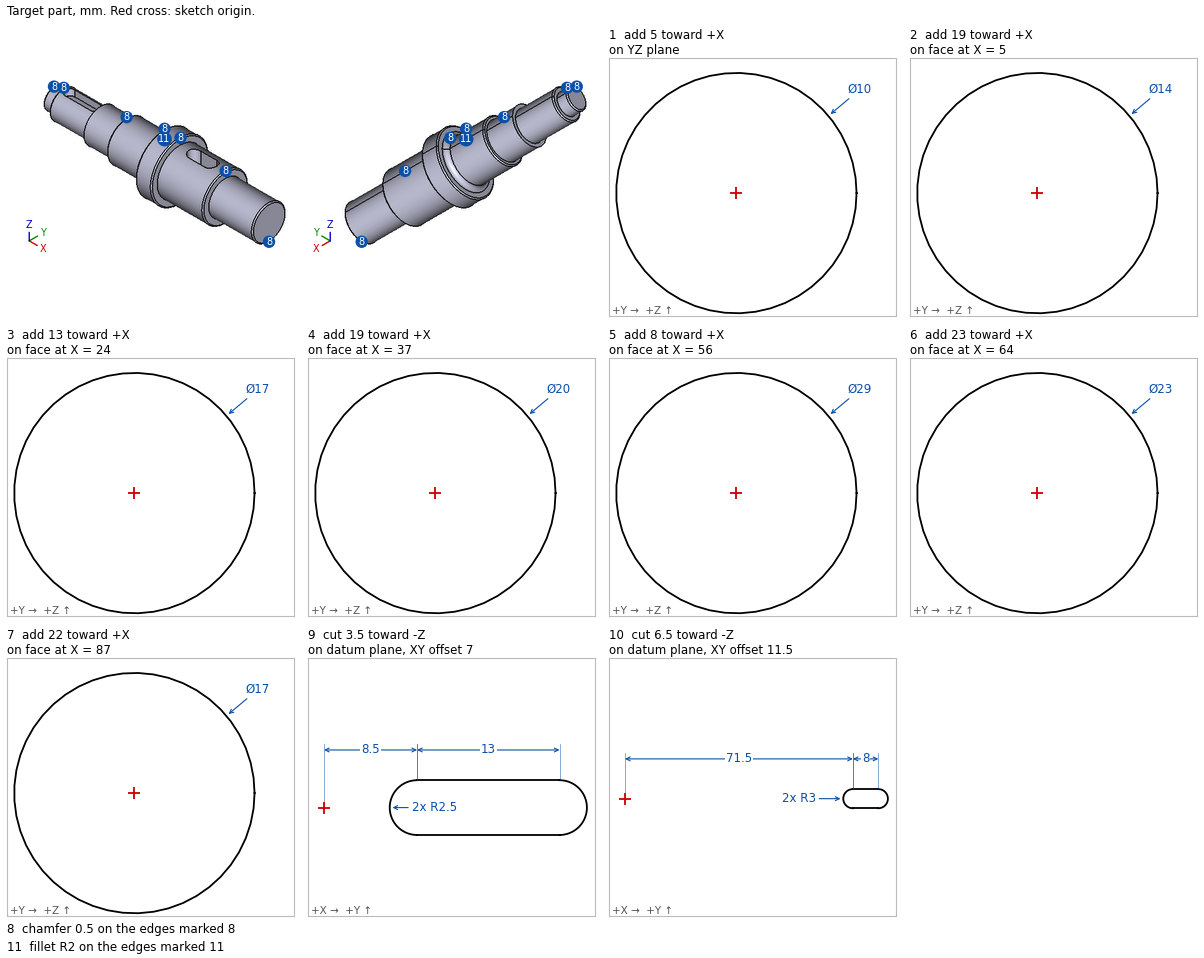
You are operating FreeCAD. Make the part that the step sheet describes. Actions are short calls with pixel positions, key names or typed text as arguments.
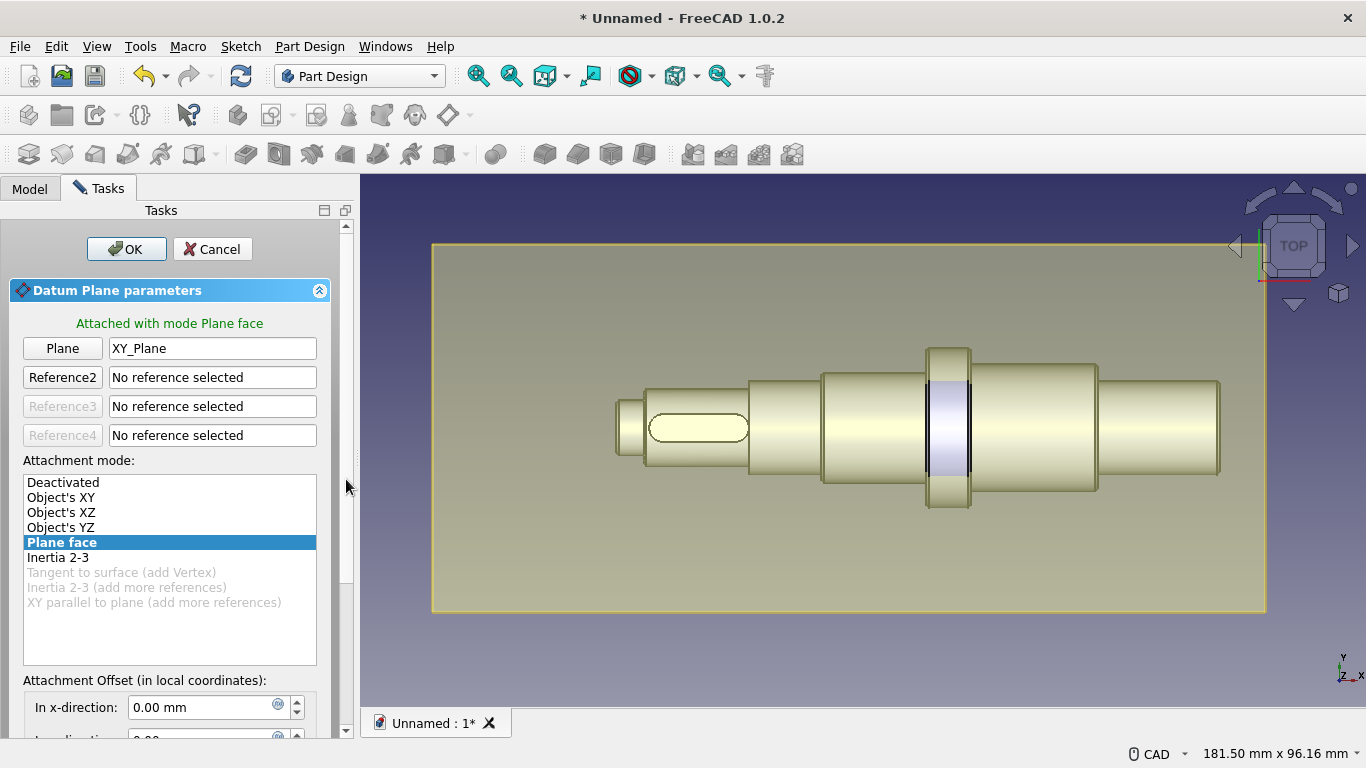
click(127, 249)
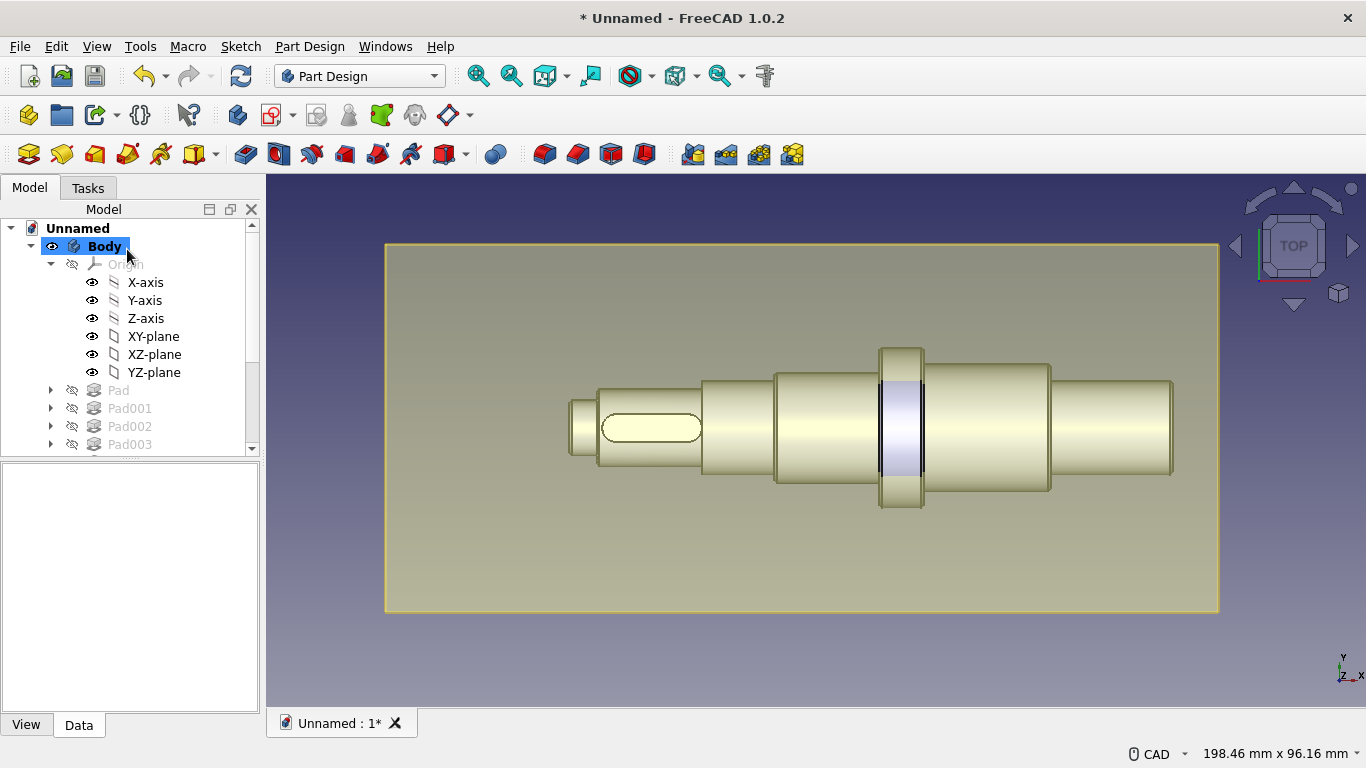
scroll(101, 332, down, 3)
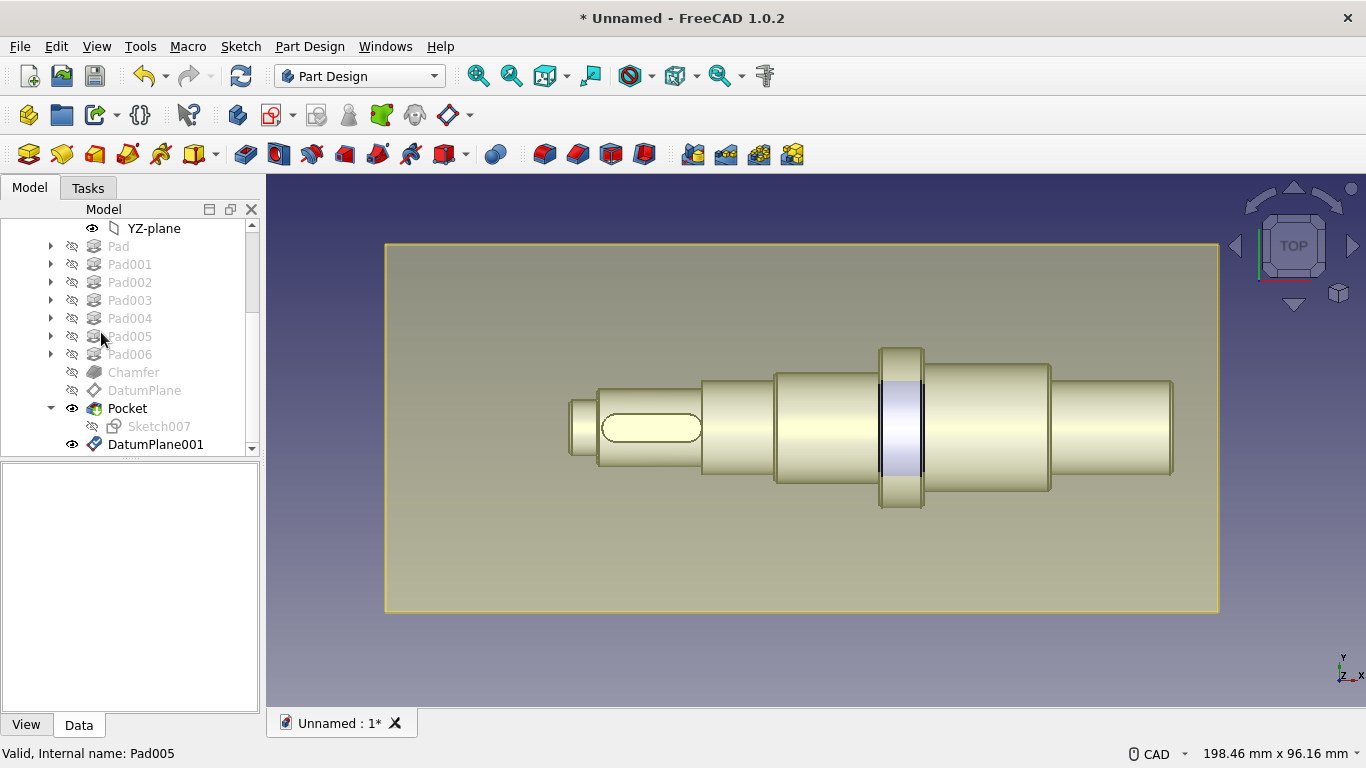
click(117, 444)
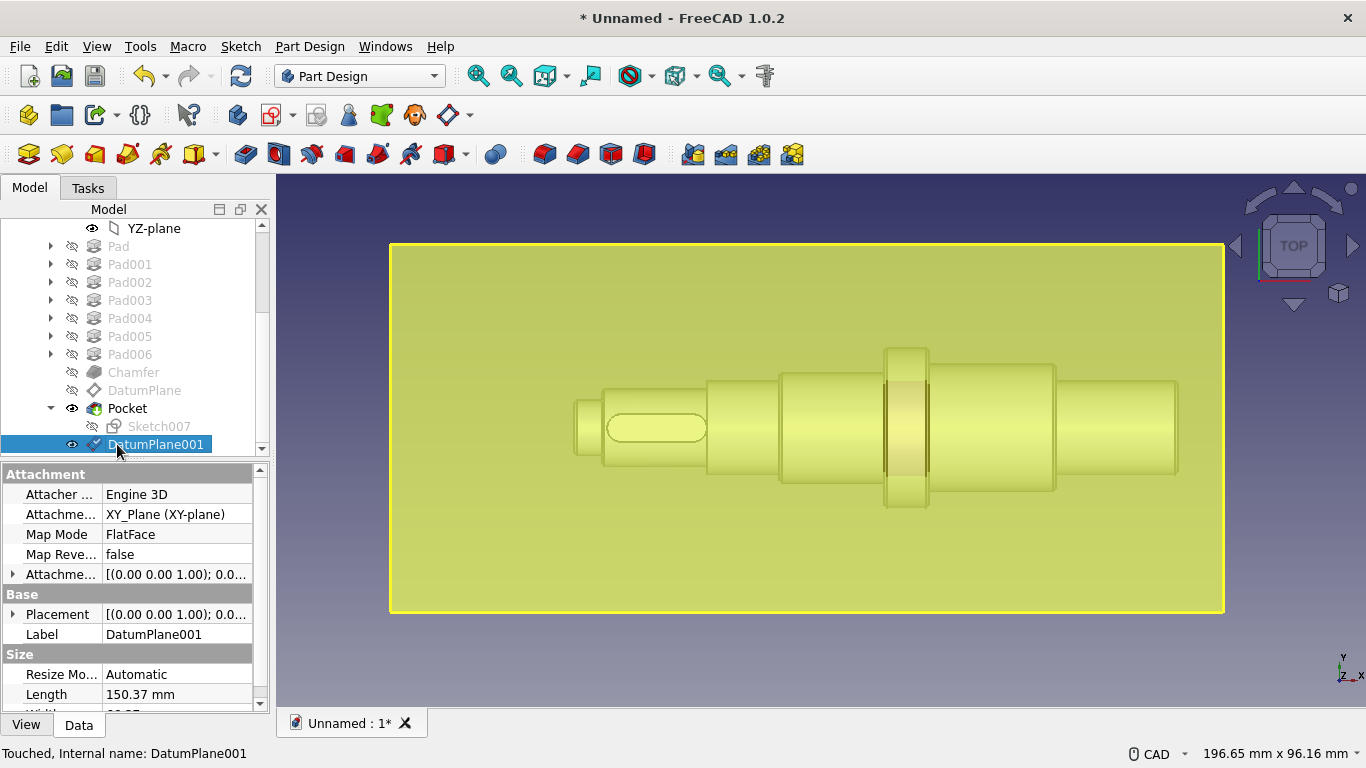
click(270, 116)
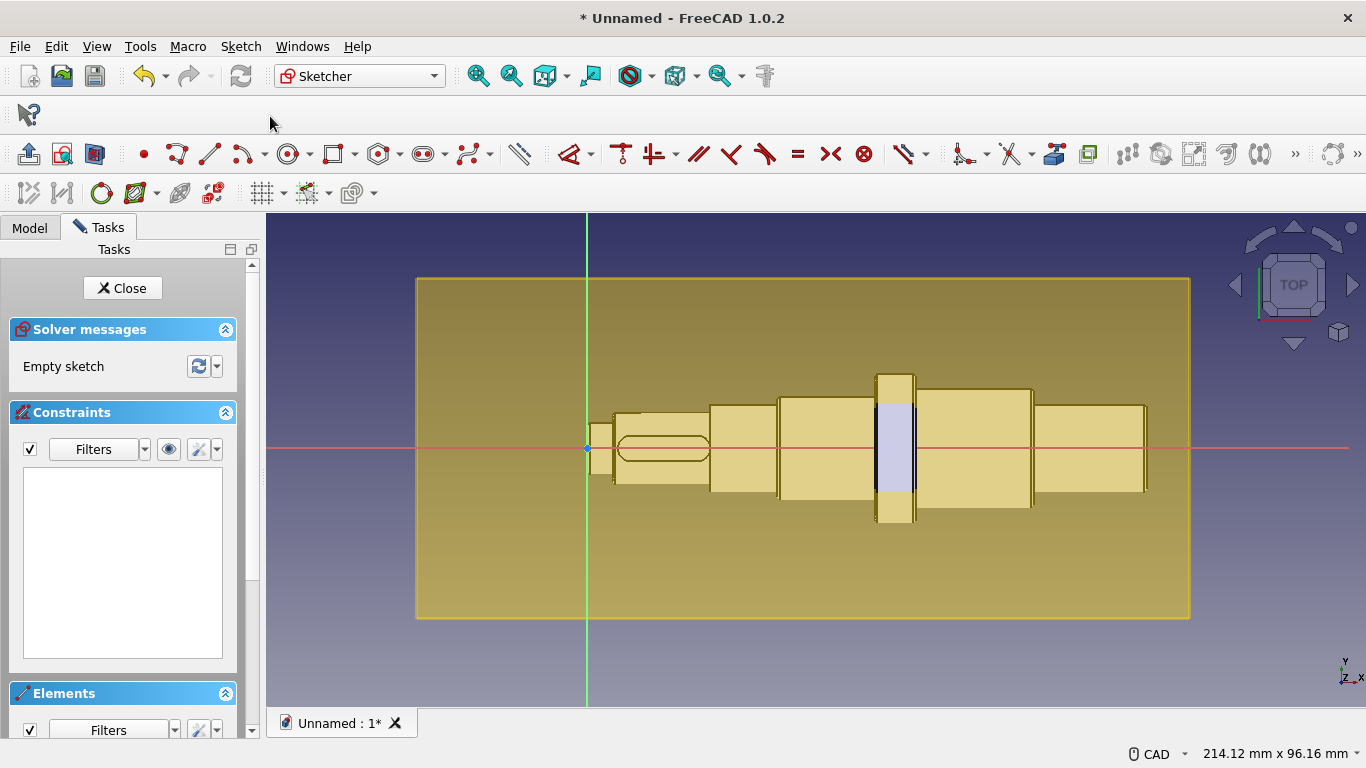
click(95, 154)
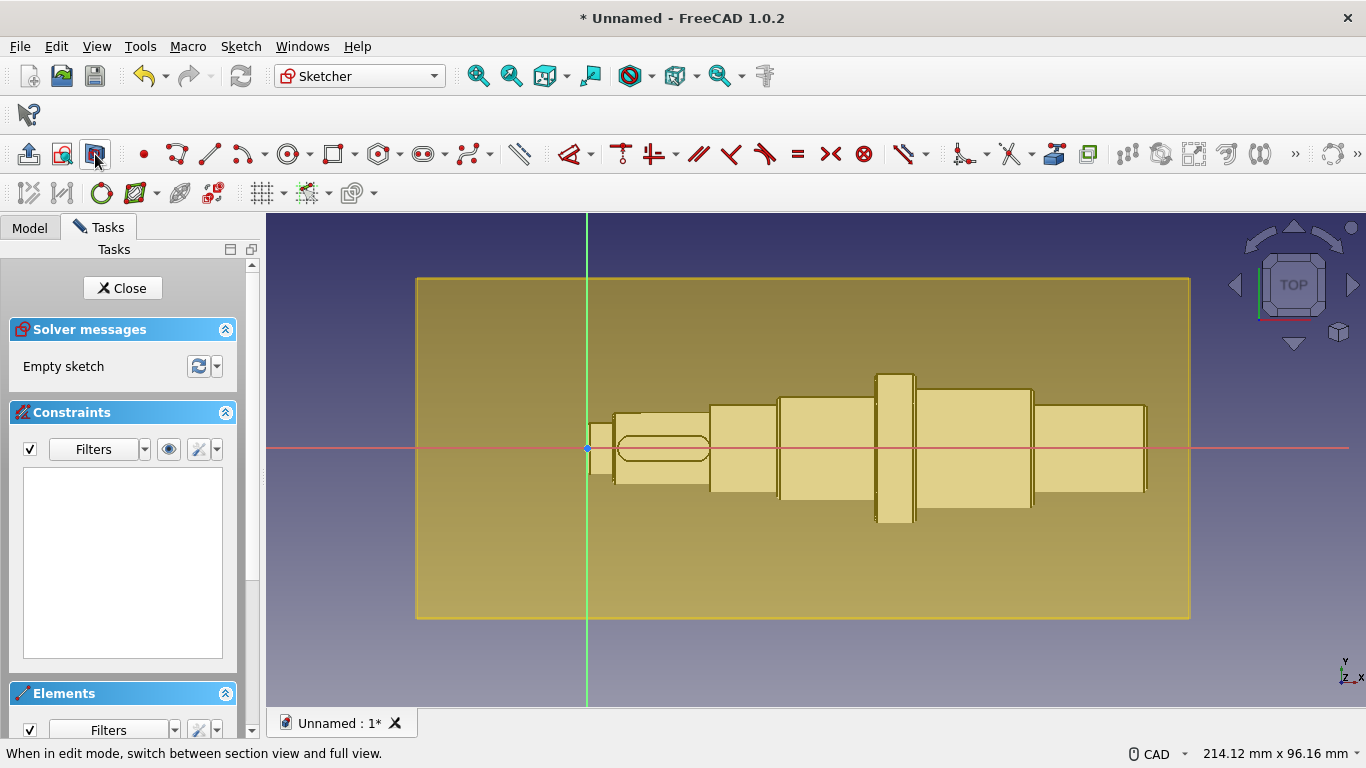
scroll(1003, 447, up, 11)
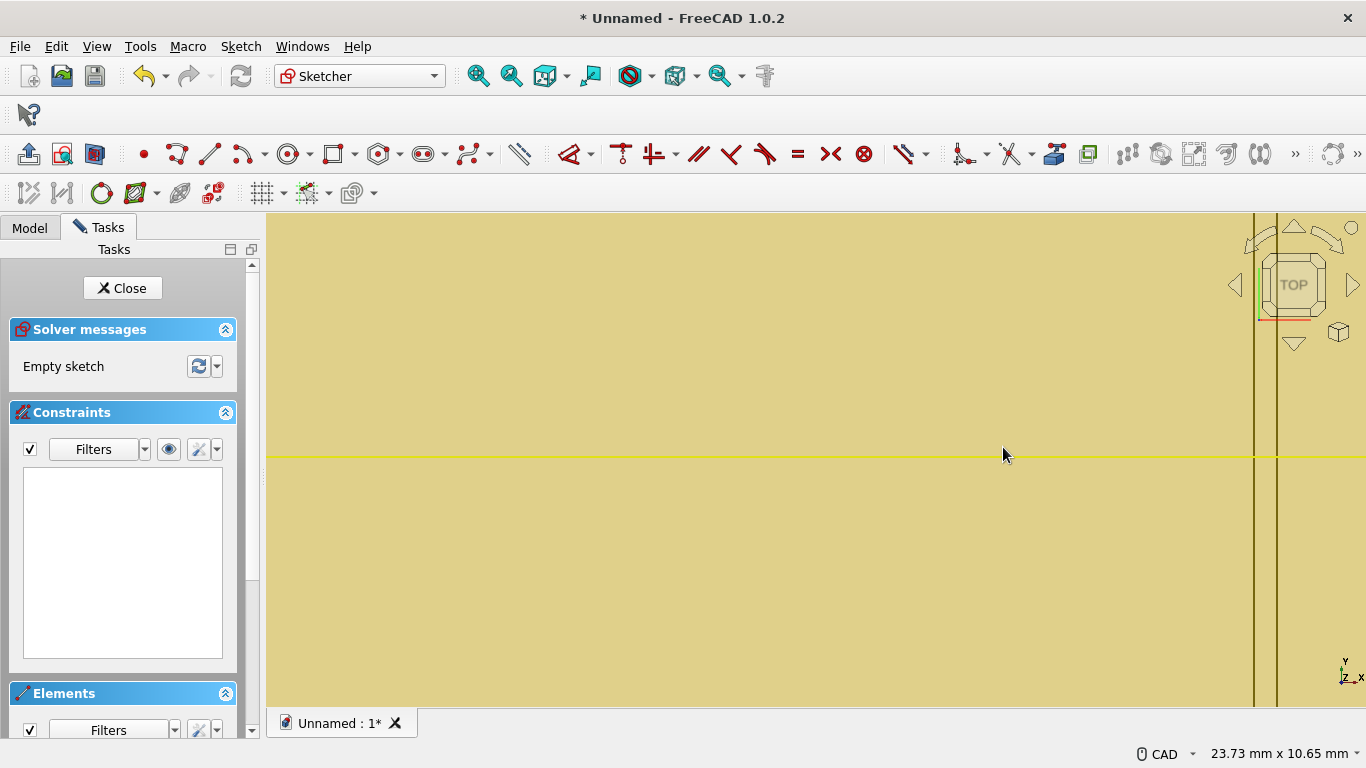
key(g)
key(s)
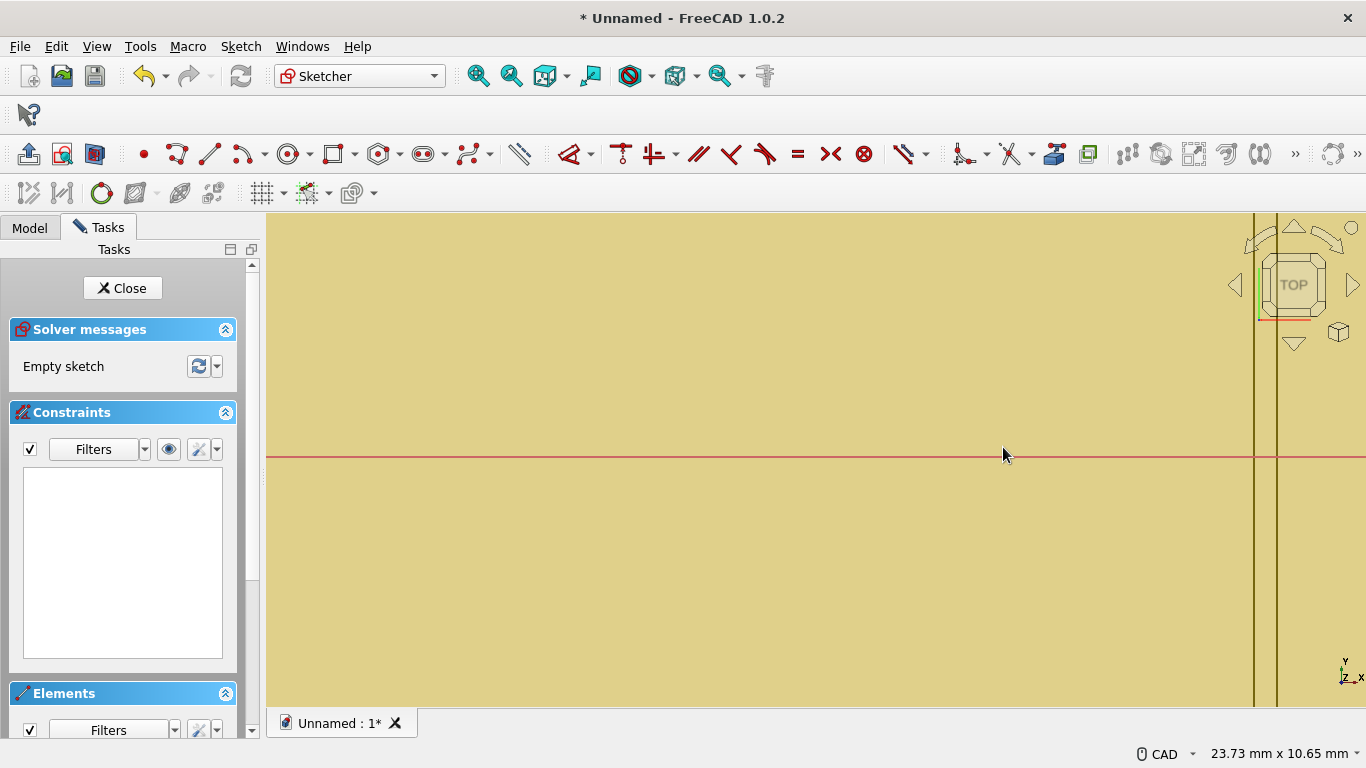
click(559, 457)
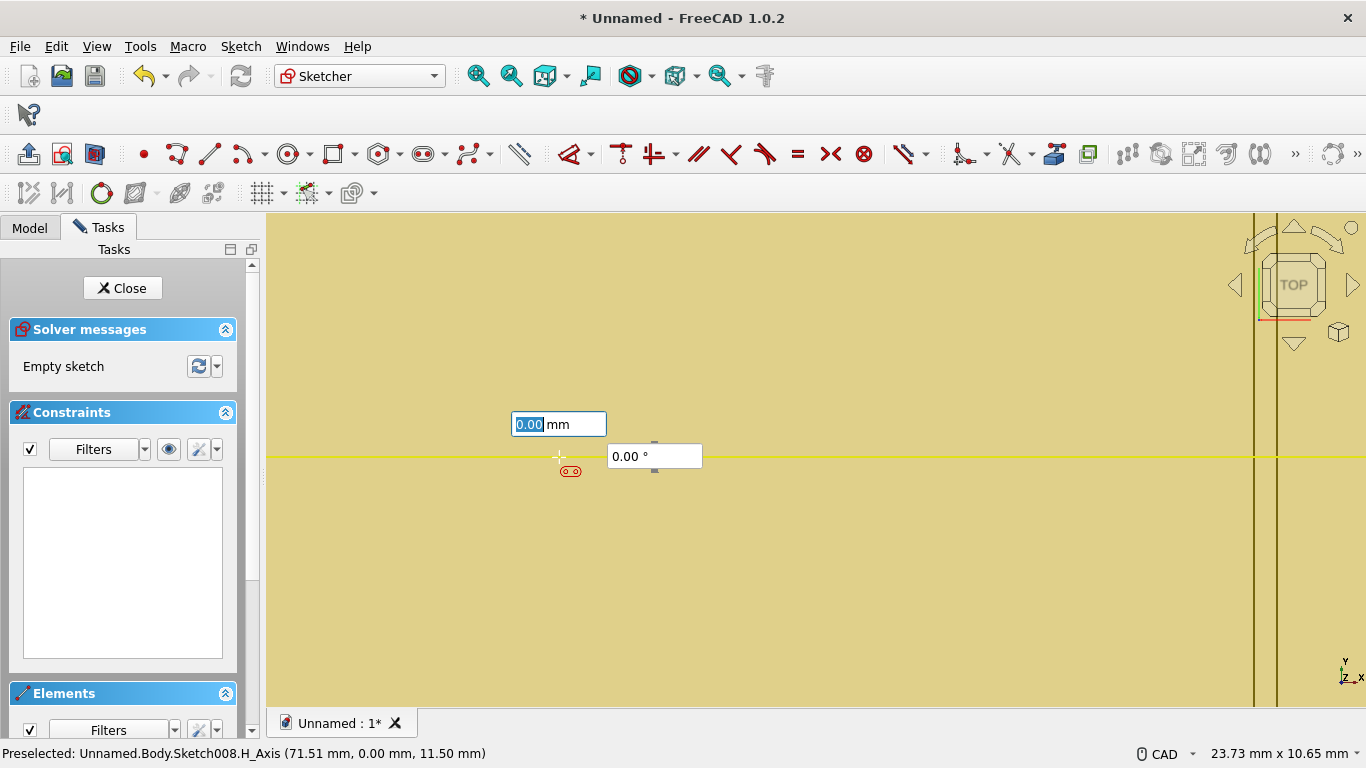
click(929, 448)